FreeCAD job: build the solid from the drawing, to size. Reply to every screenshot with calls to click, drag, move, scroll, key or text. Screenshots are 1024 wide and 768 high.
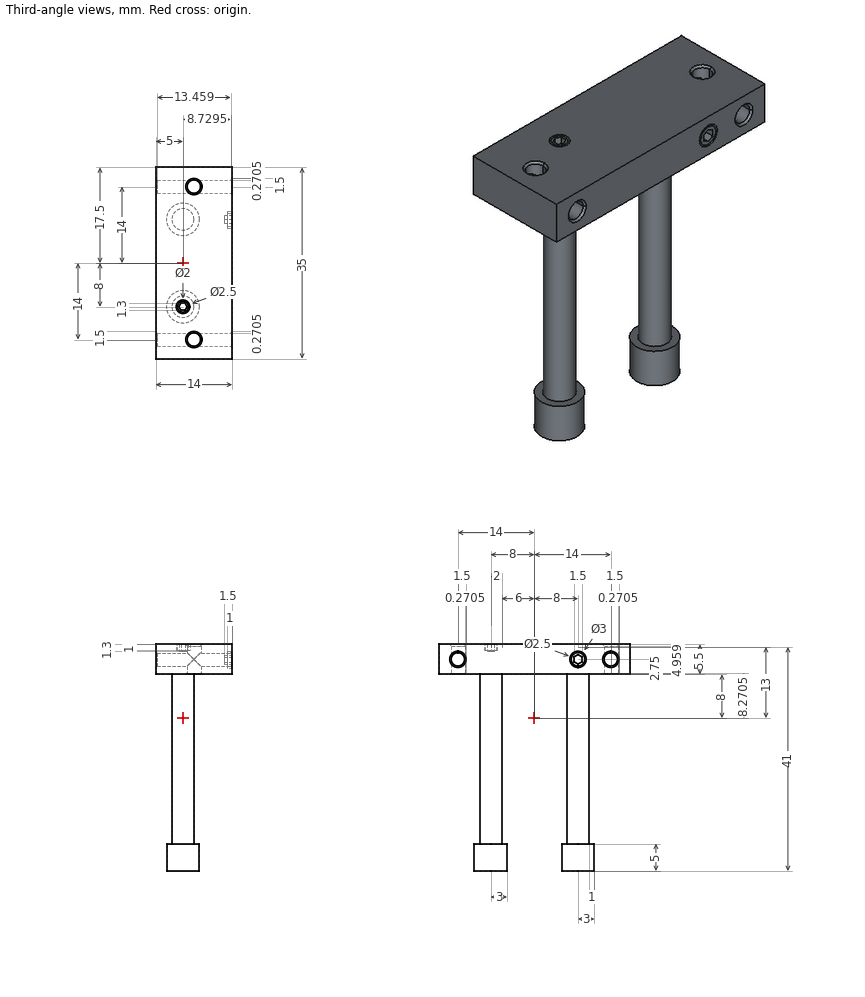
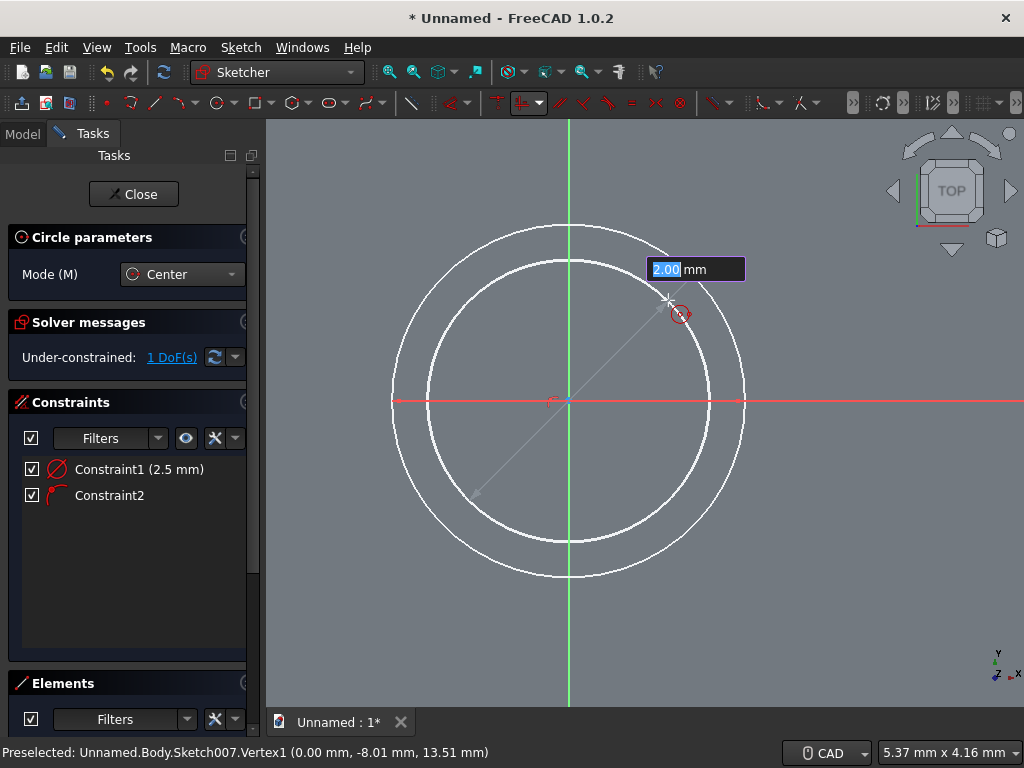
text(2)
key(Return)
key(Escape)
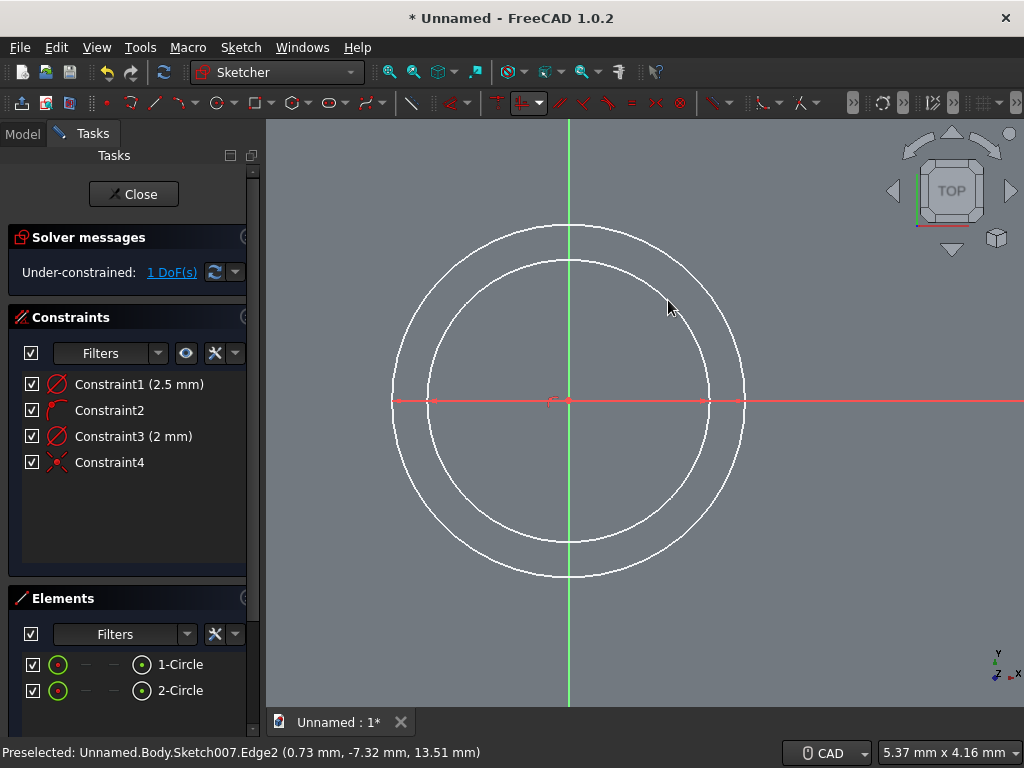
click(450, 104)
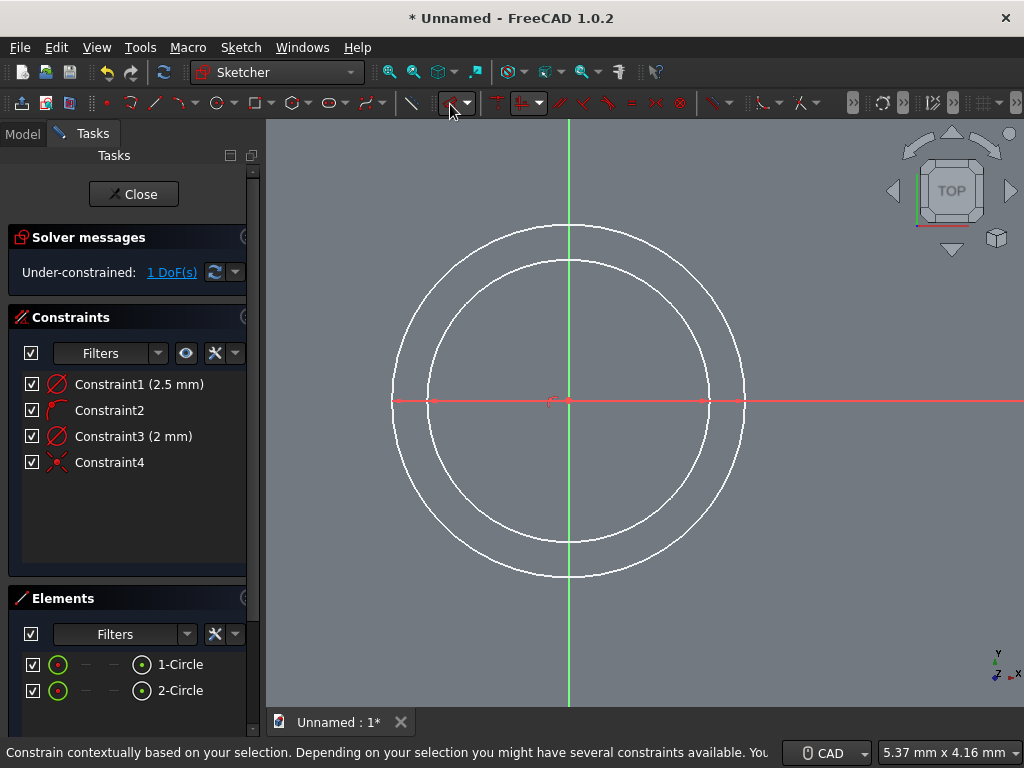
click(569, 401)
click(603, 332)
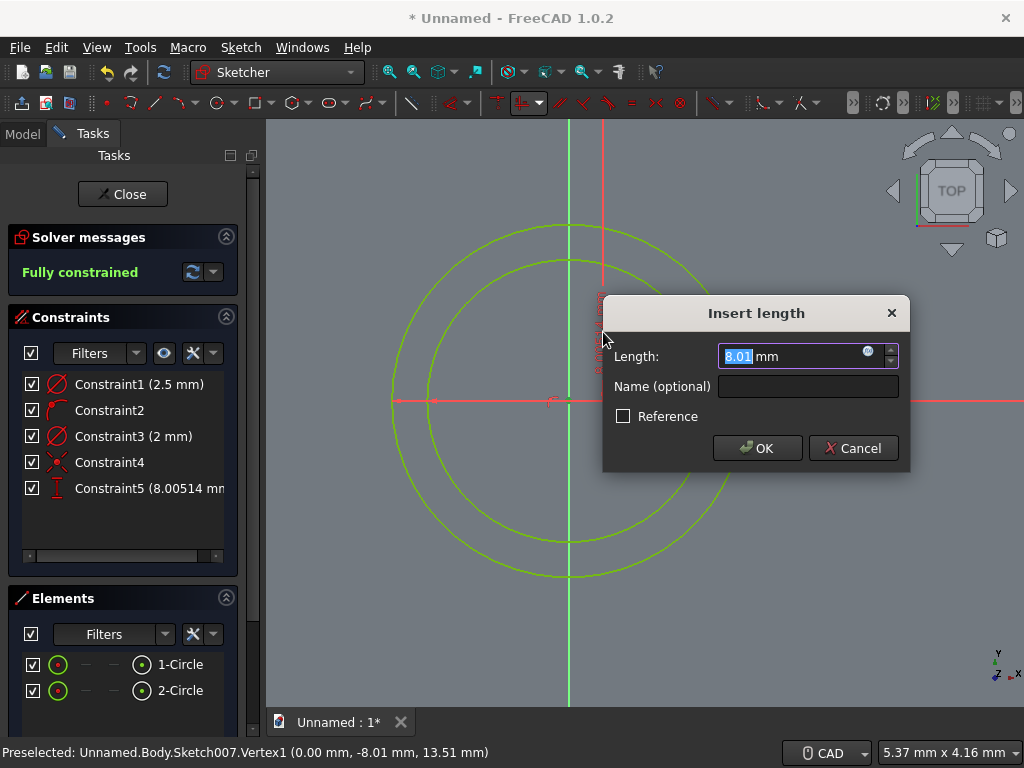
text(8)
key(Return)
key(Escape)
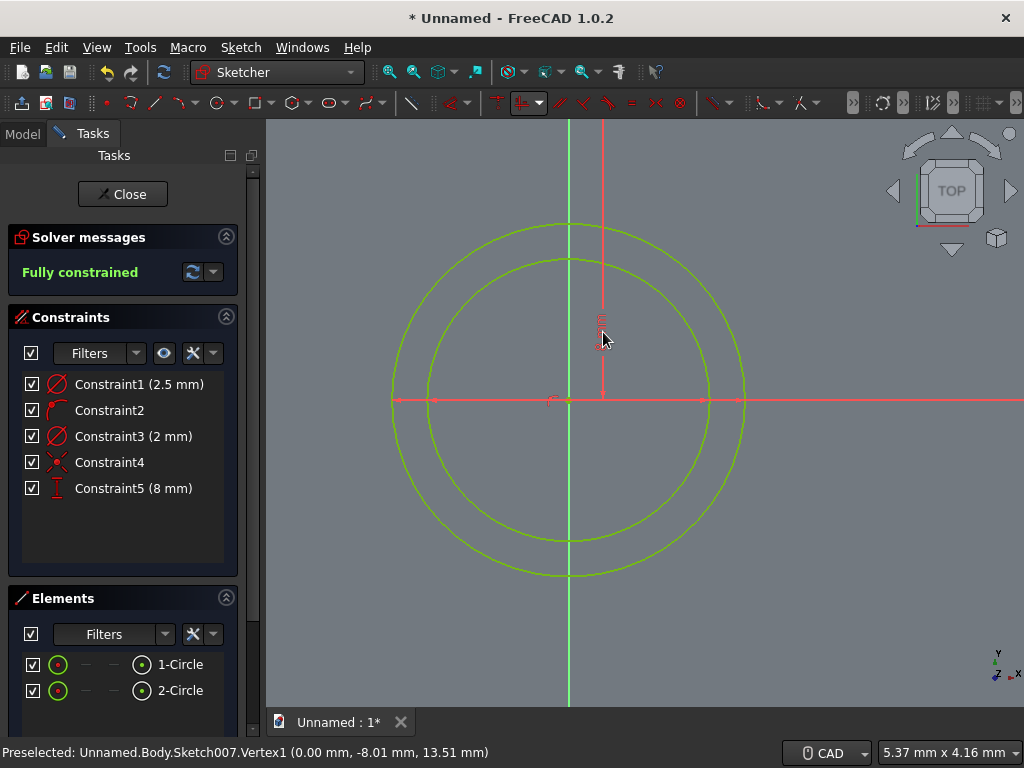
click(123, 194)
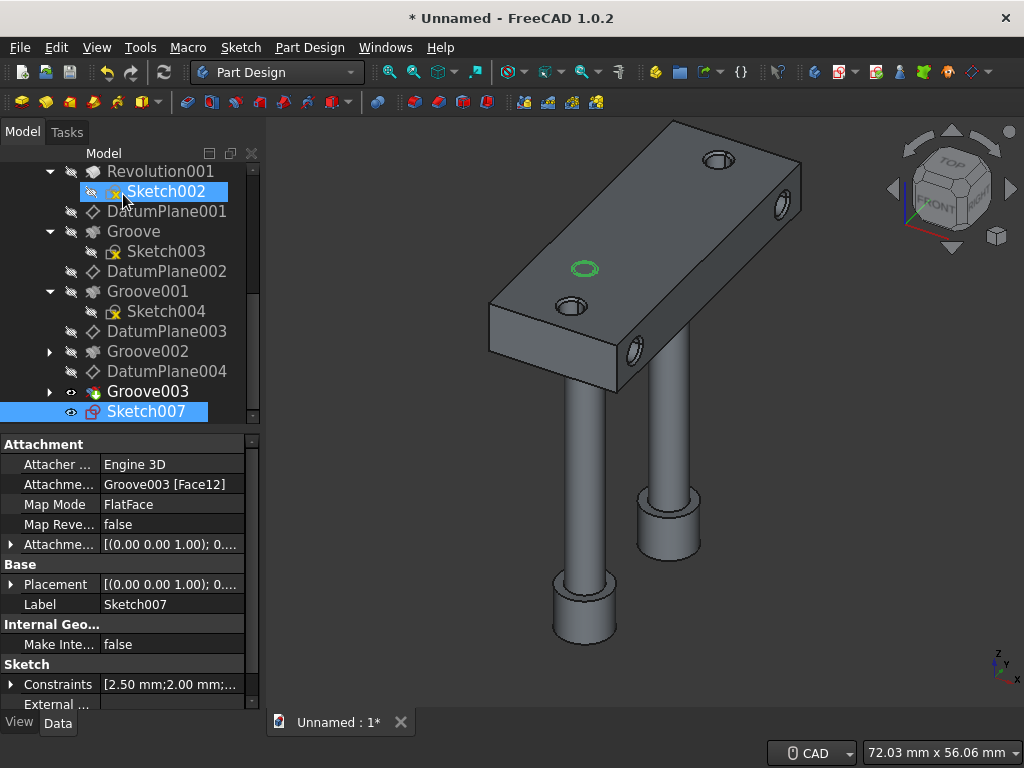
click(188, 102)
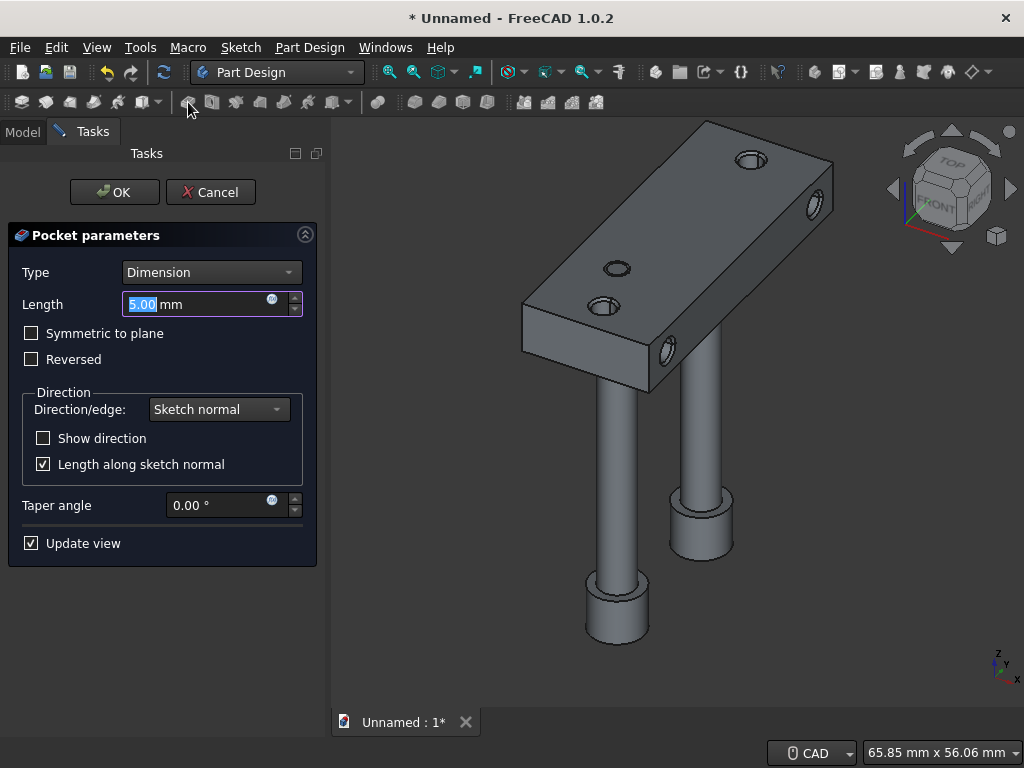
text(1)
key(Tab)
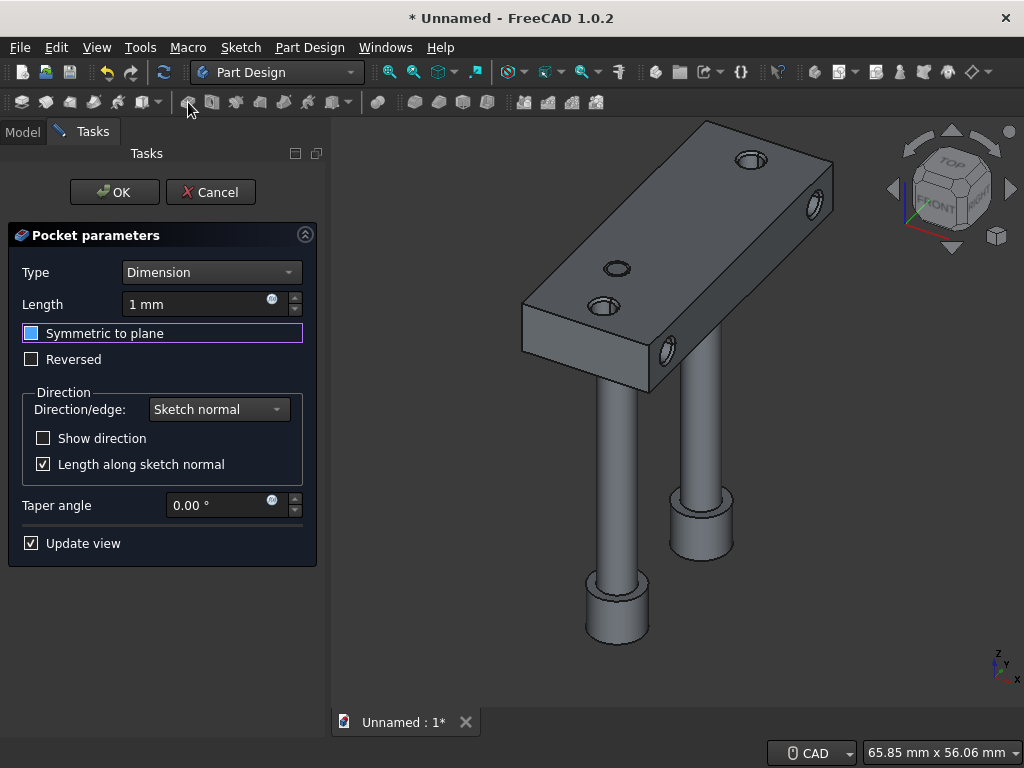
click(115, 192)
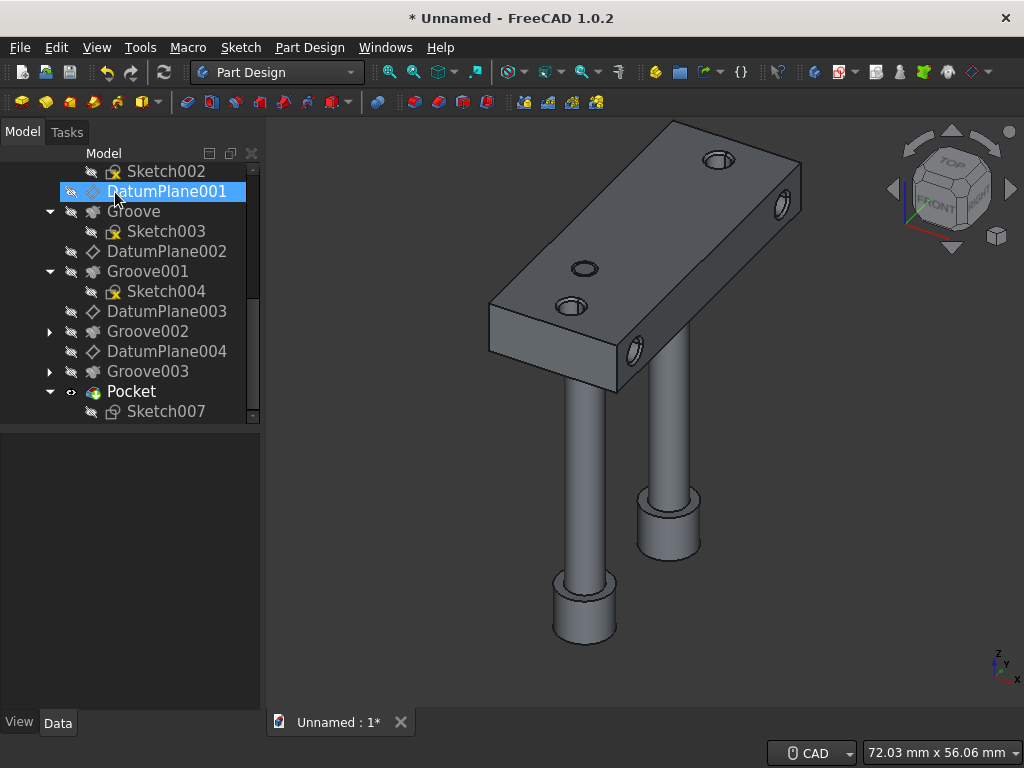
click(671, 206)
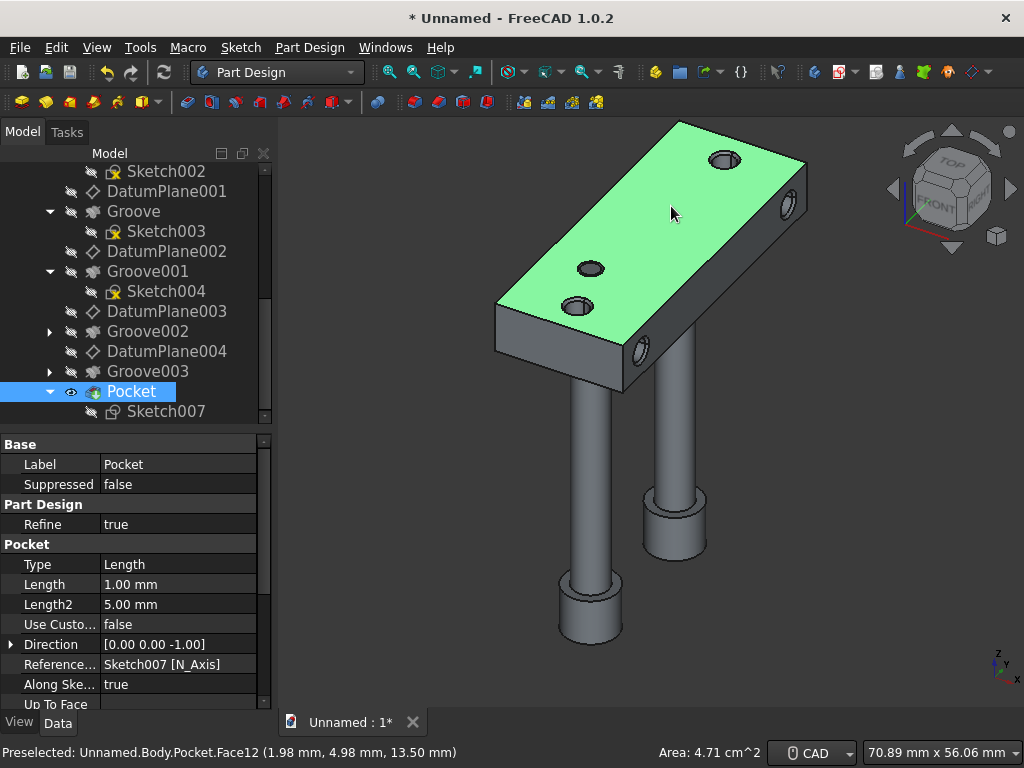
click(840, 72)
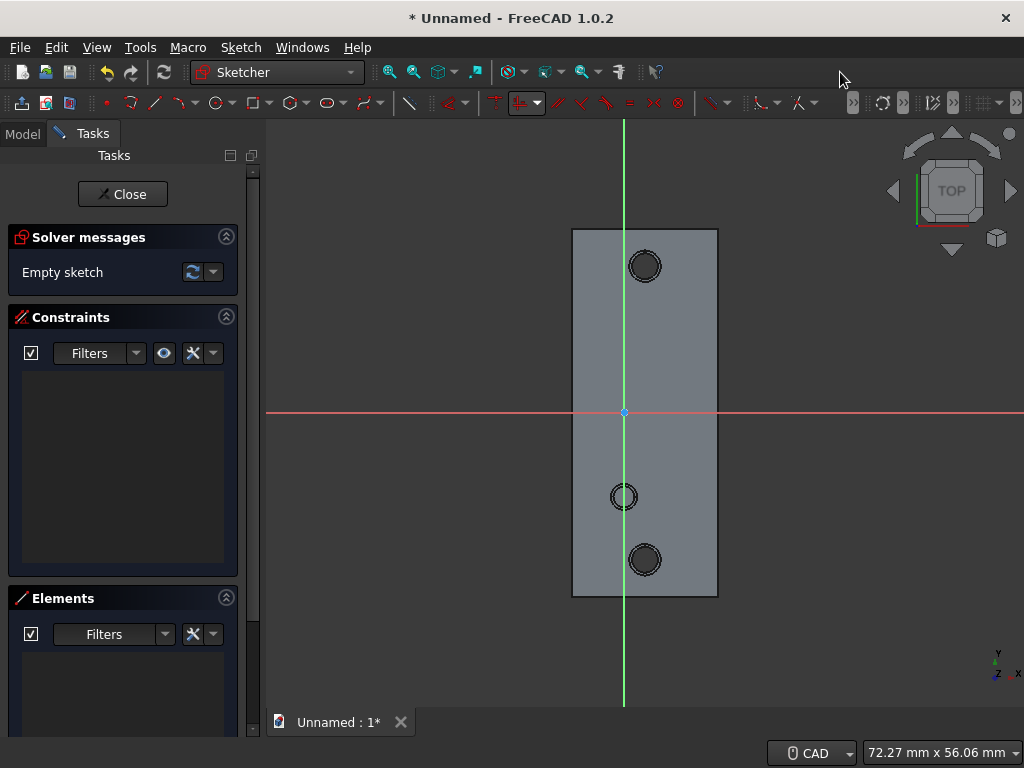
scroll(627, 501, up, 15)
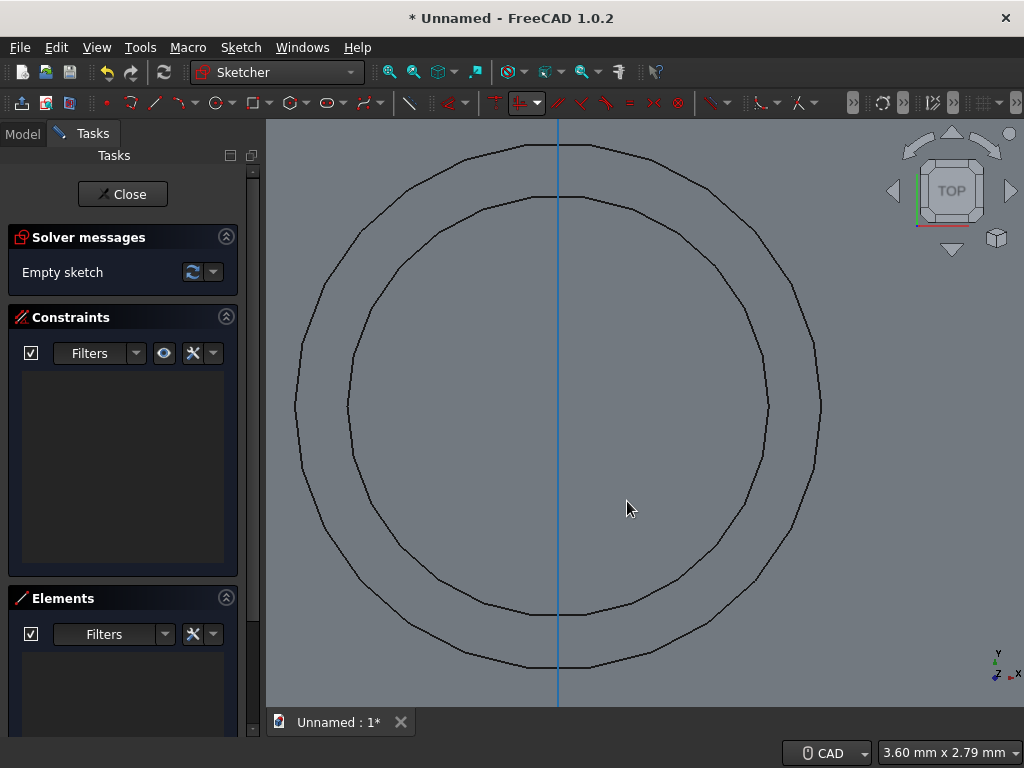
click(290, 104)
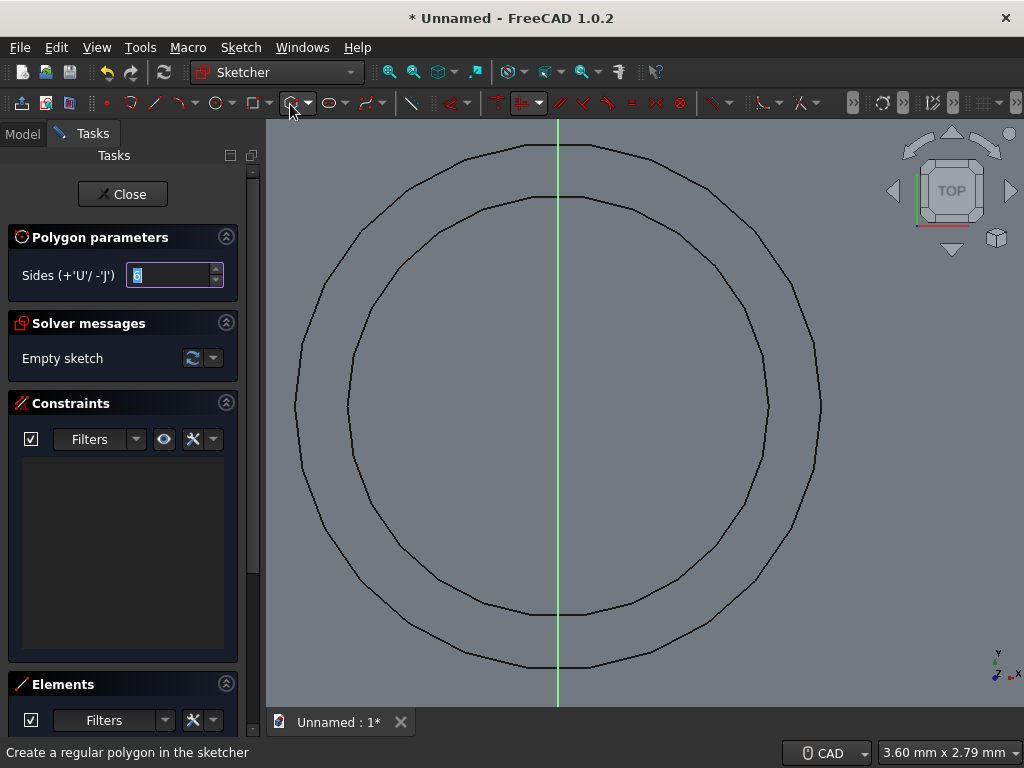
click(558, 406)